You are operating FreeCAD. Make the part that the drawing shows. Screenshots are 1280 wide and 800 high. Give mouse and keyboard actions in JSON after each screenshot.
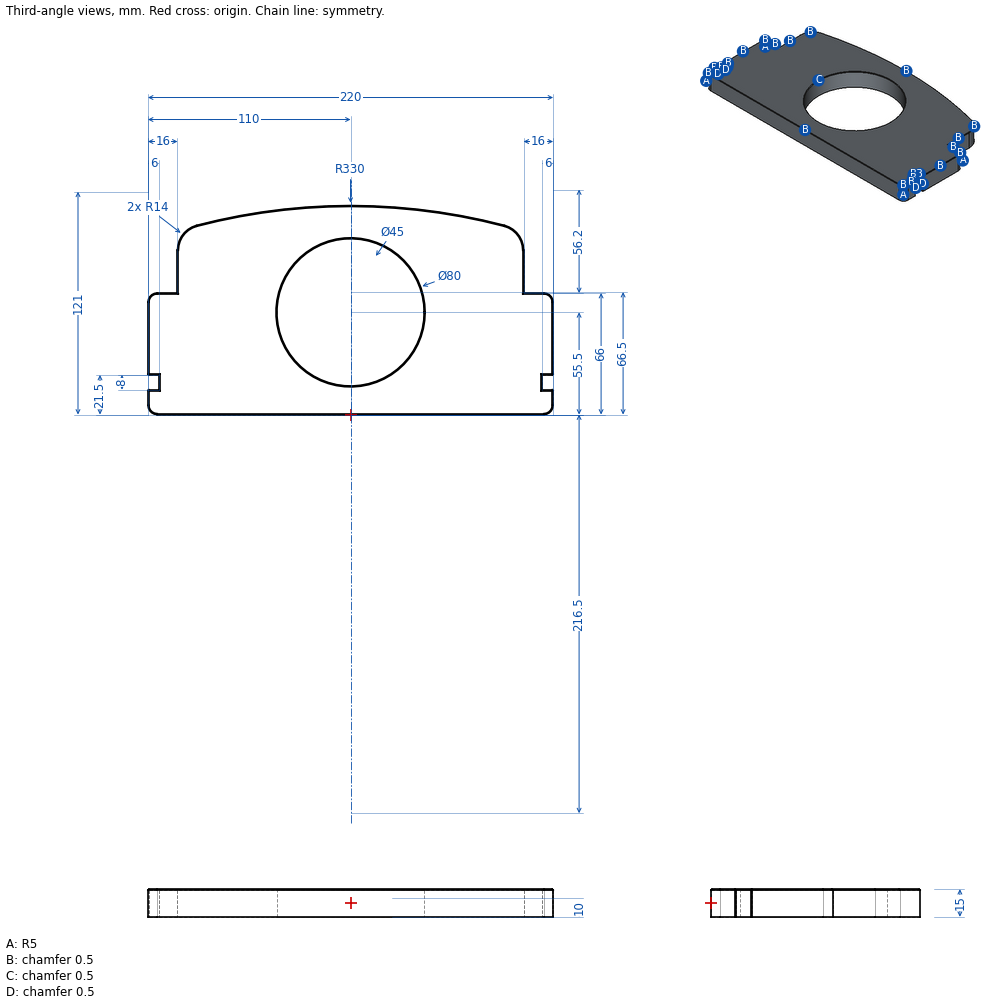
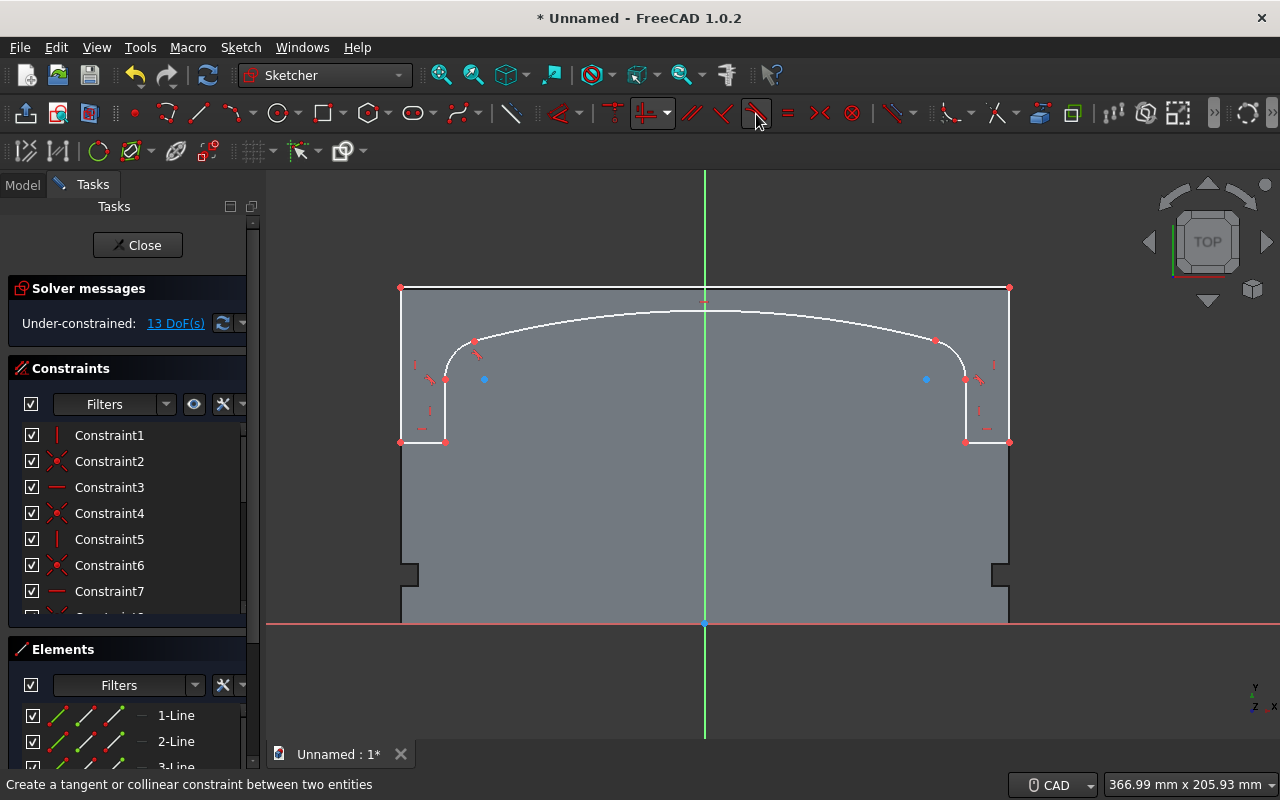
{"action": "left_click", "coordinate": [798, 316]}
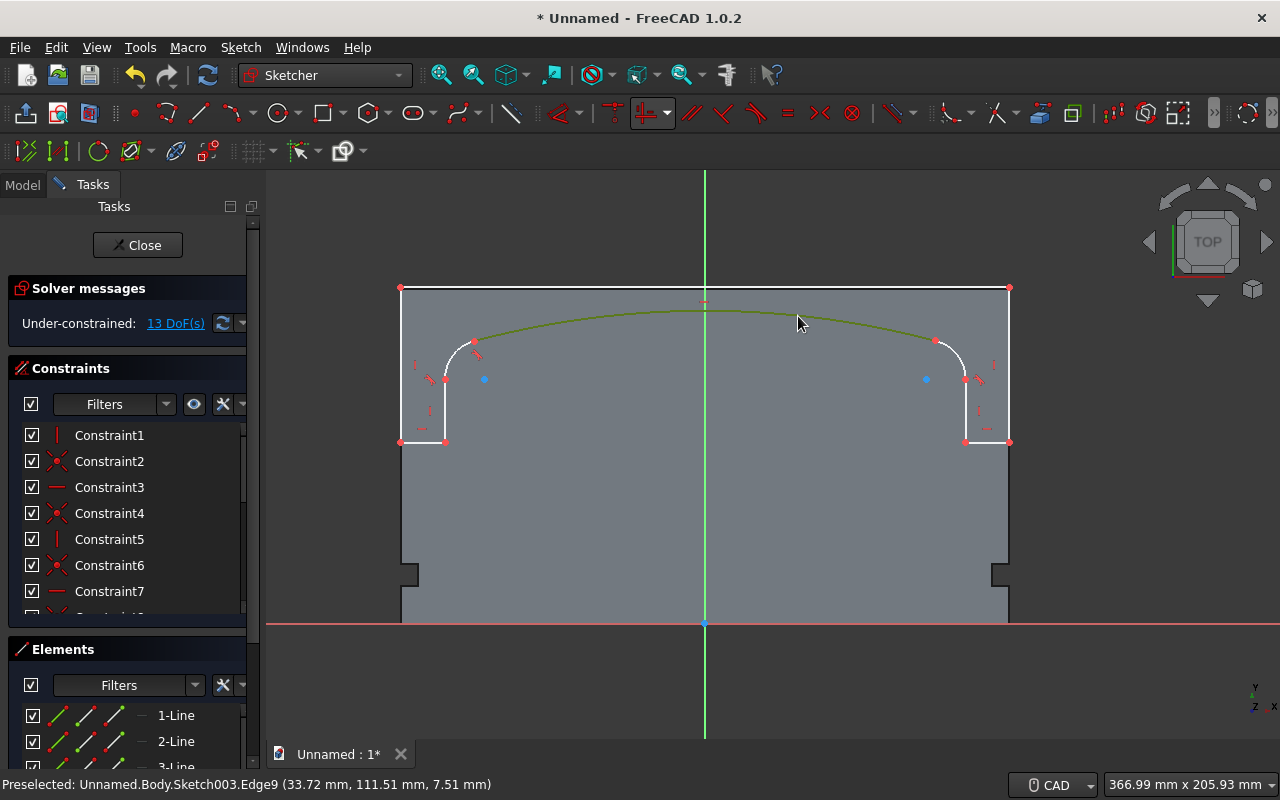
{"action": "left_click", "coordinate": [962, 364]}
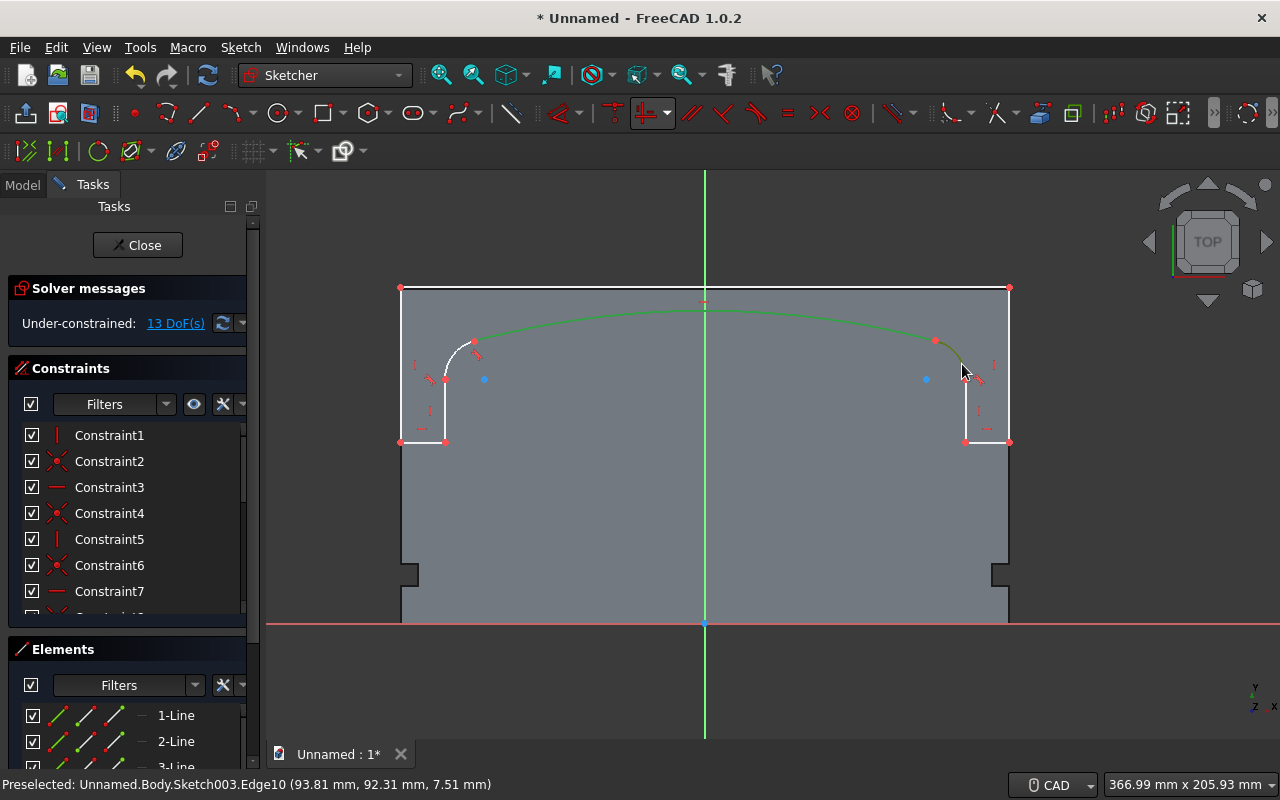
{"action": "left_click", "coordinate": [756, 114]}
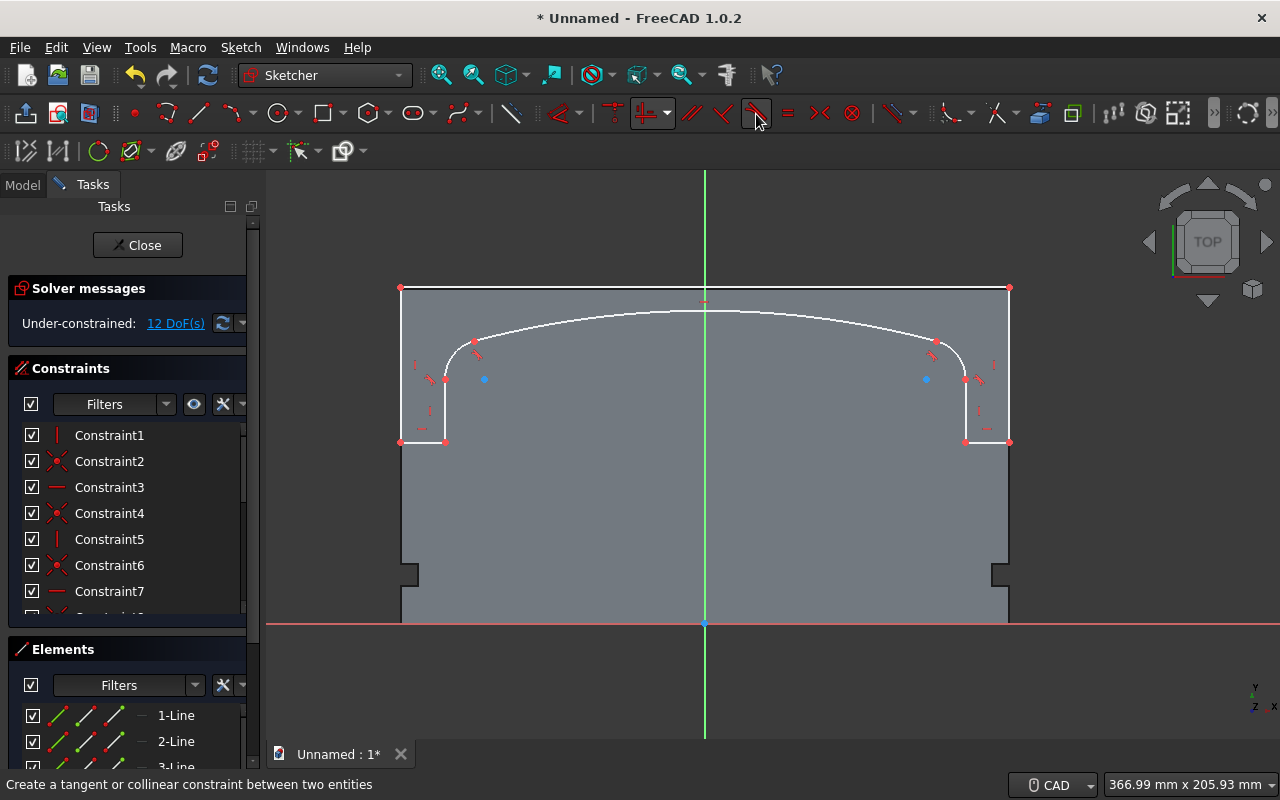
{"action": "left_click", "coordinate": [460, 348]}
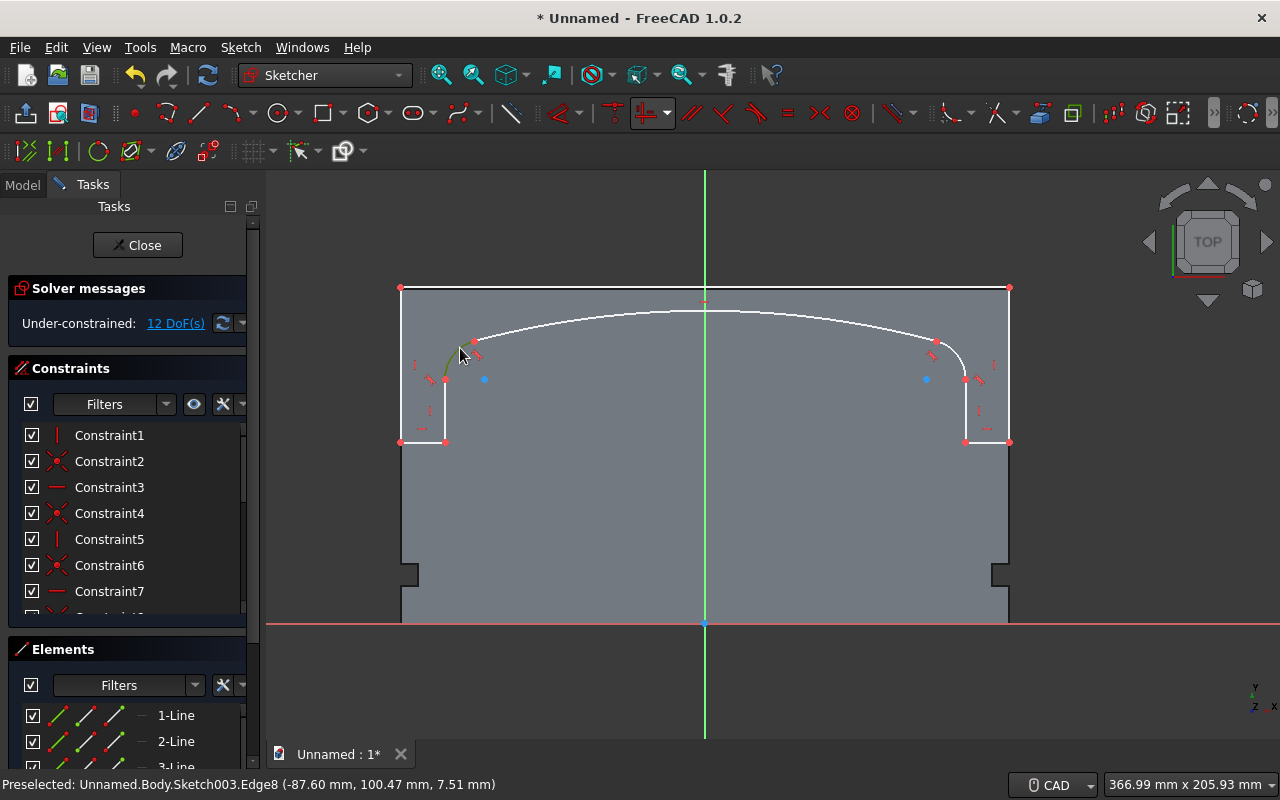
{"action": "left_click", "coordinate": [963, 364]}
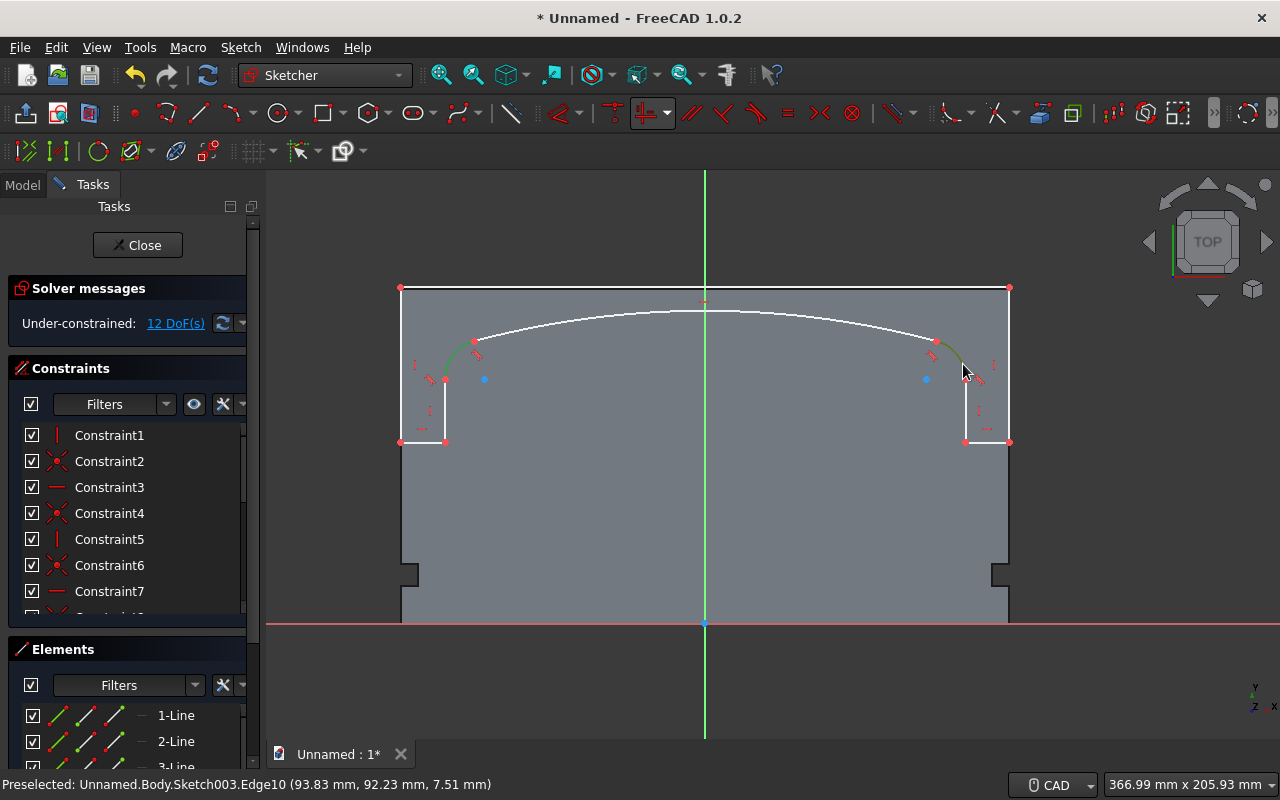
{"action": "left_click", "coordinate": [788, 114]}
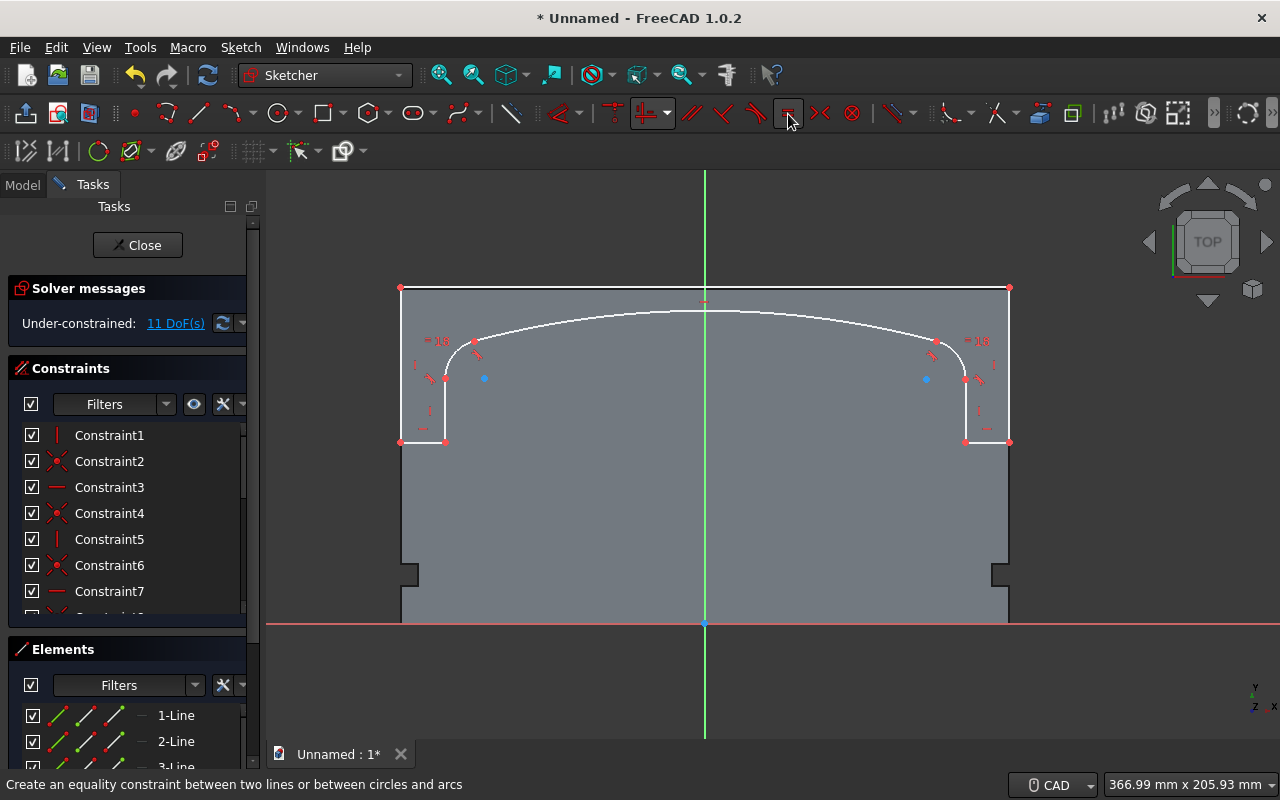
{"action": "scroll", "coordinate": [704, 285], "scroll_direction": "down", "scroll_amount": 5}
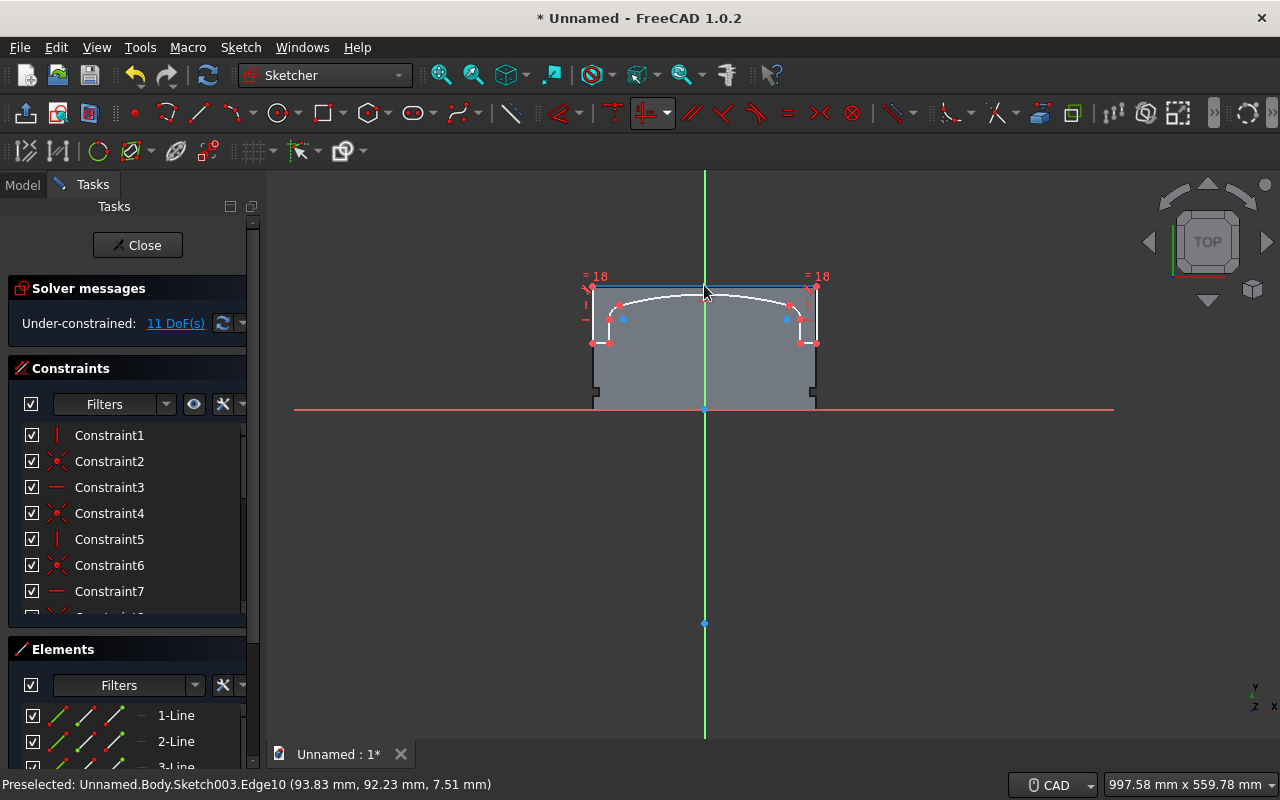
{"action": "left_click", "coordinate": [705, 623]}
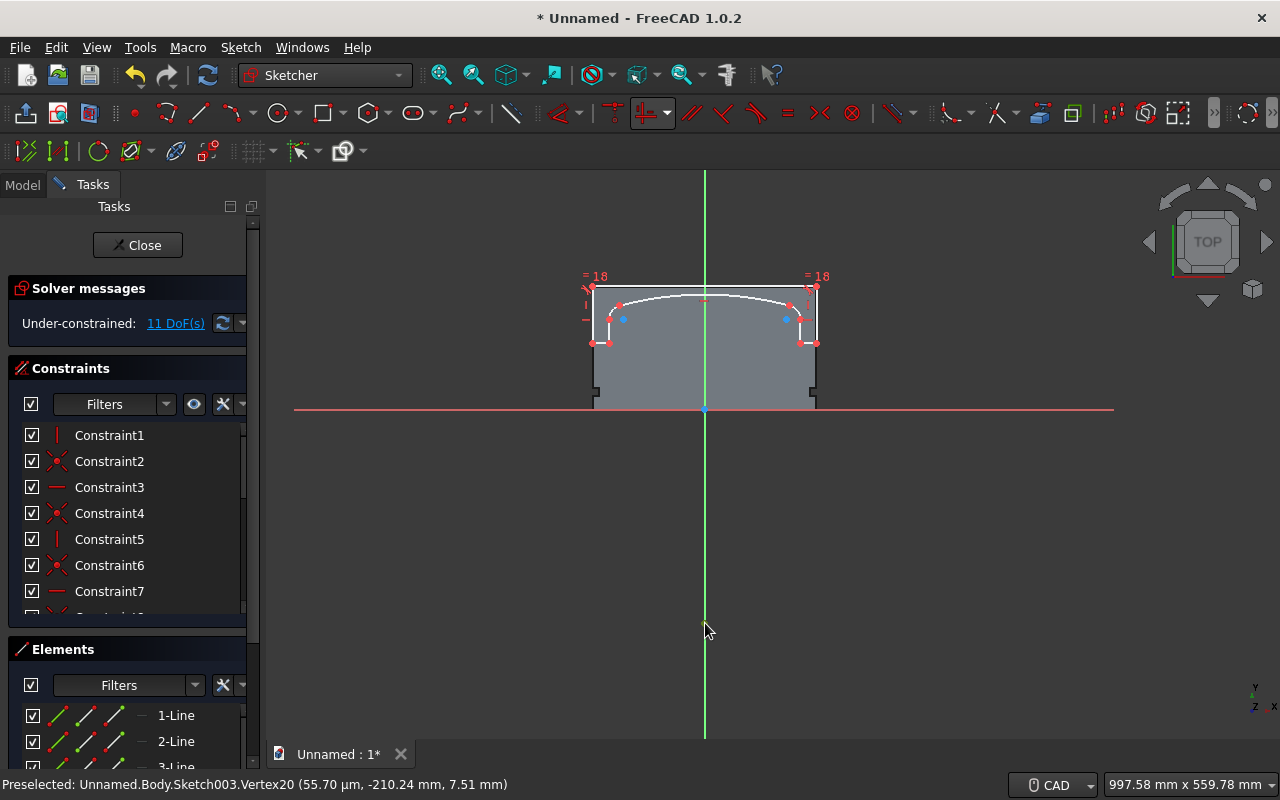
{"action": "left_click", "coordinate": [705, 674]}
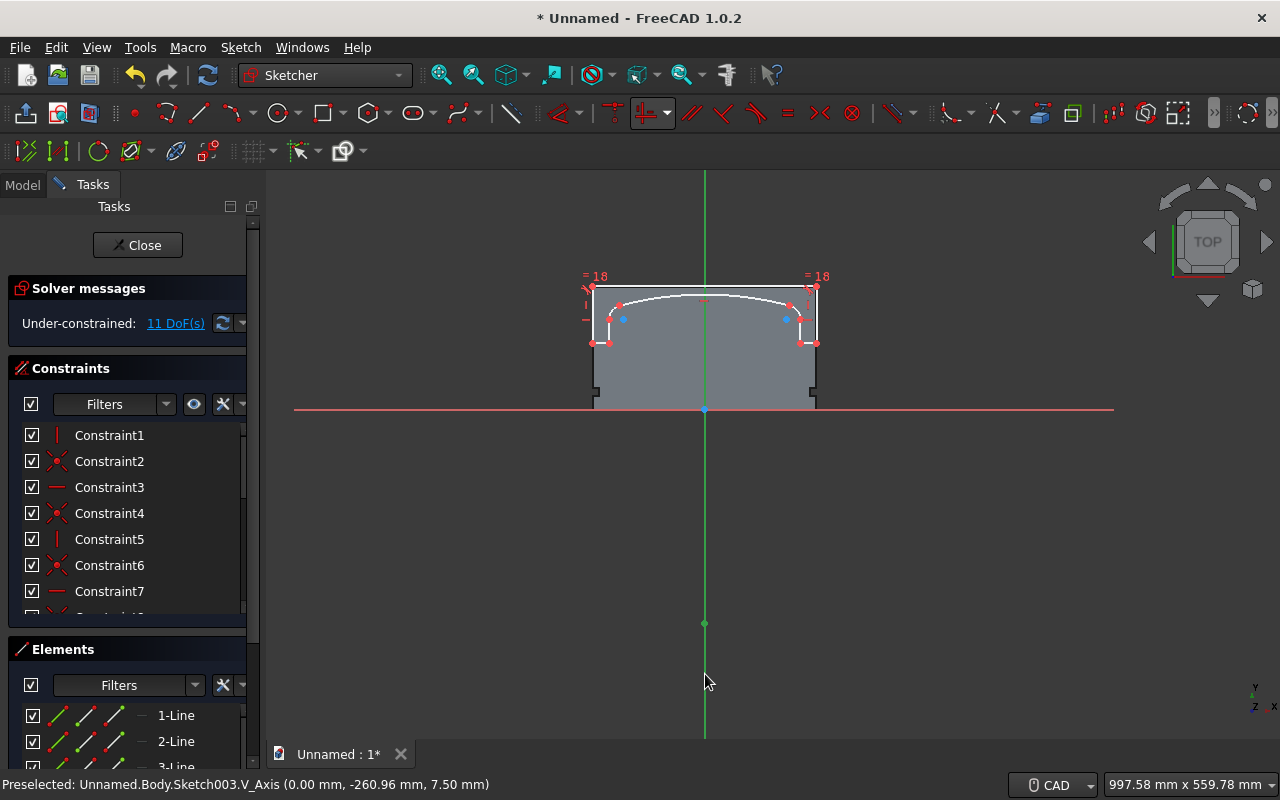
{"action": "left_click", "coordinate": [614, 114]}